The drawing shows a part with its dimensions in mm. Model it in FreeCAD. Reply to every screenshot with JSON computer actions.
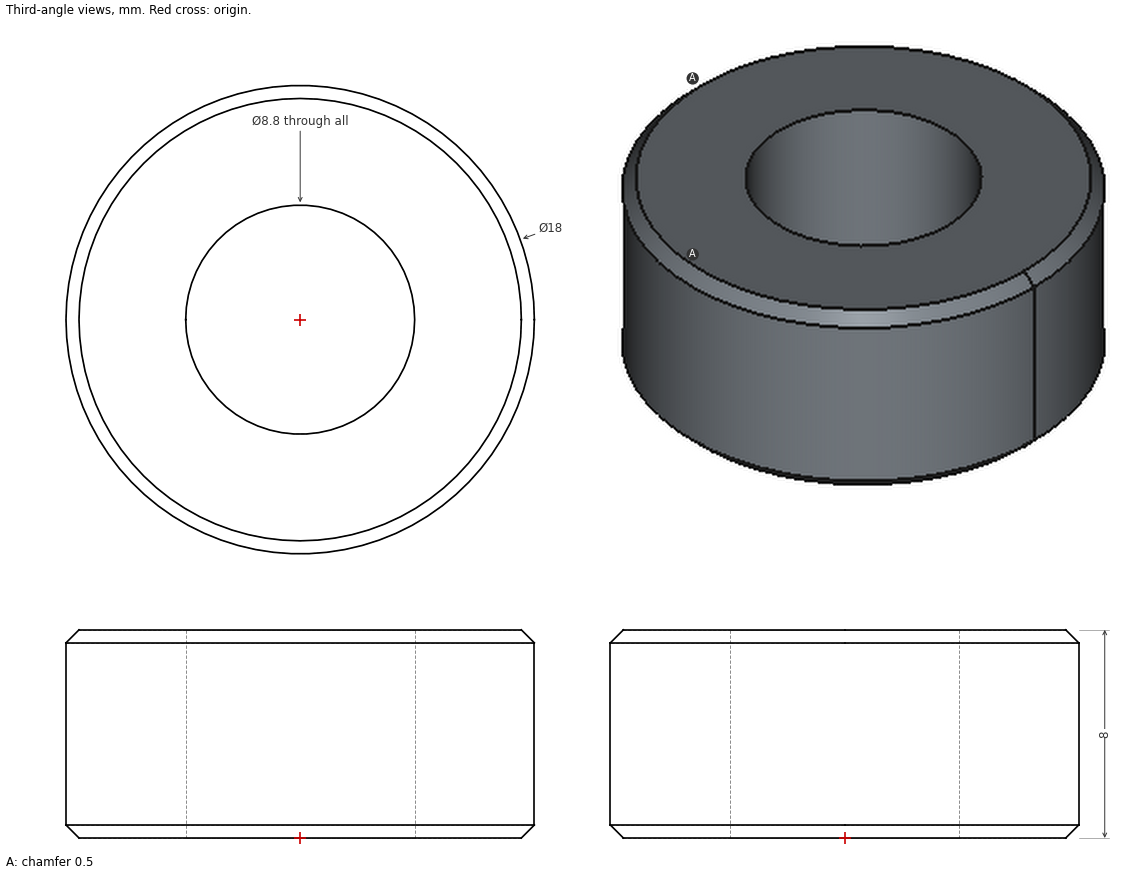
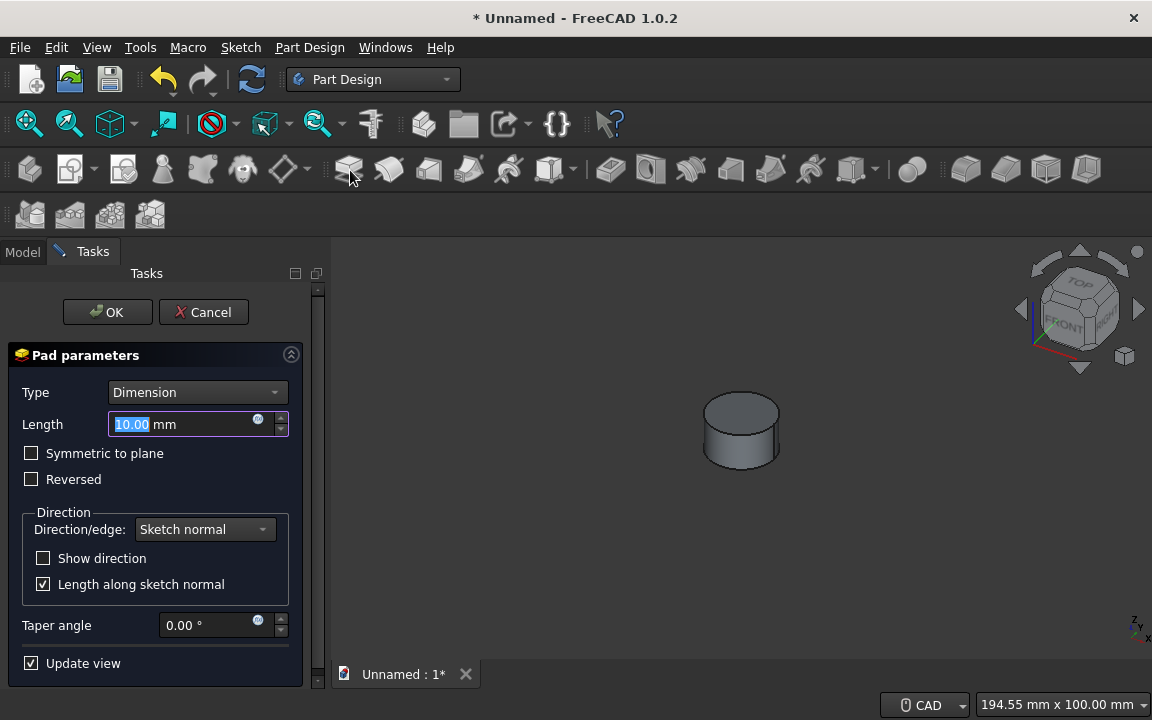
{"action": "type", "text": "8"}
{"action": "key", "text": "Tab"}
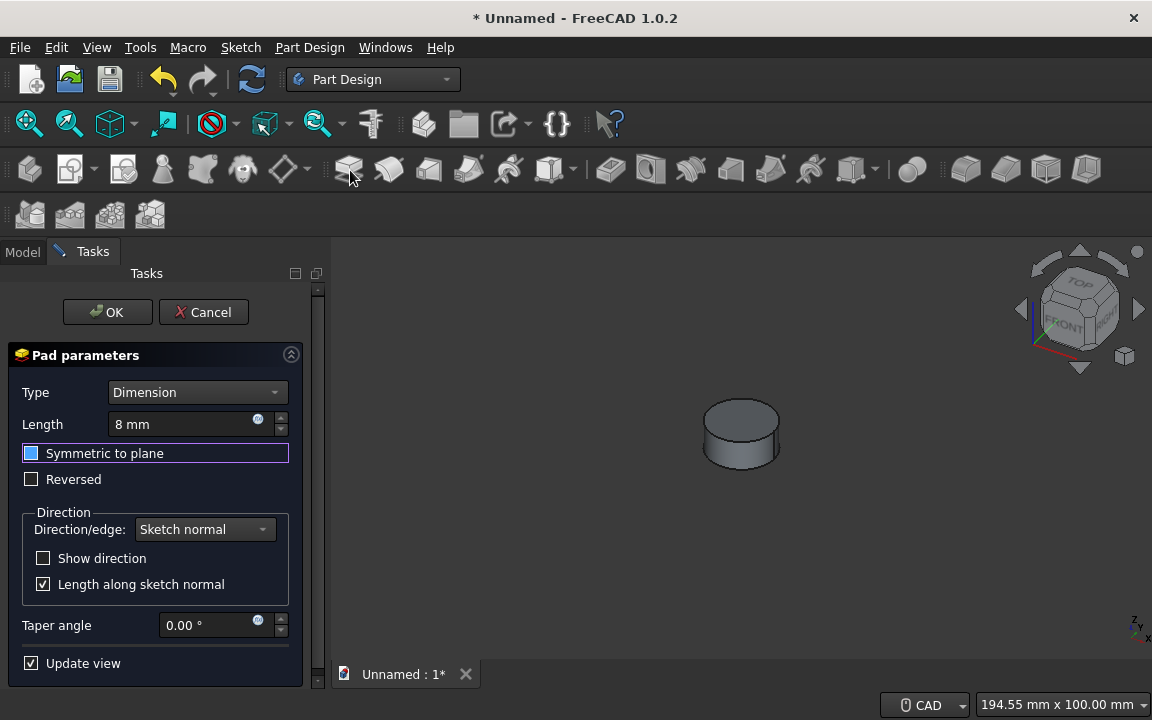
{"action": "left_click", "coordinate": [108, 312]}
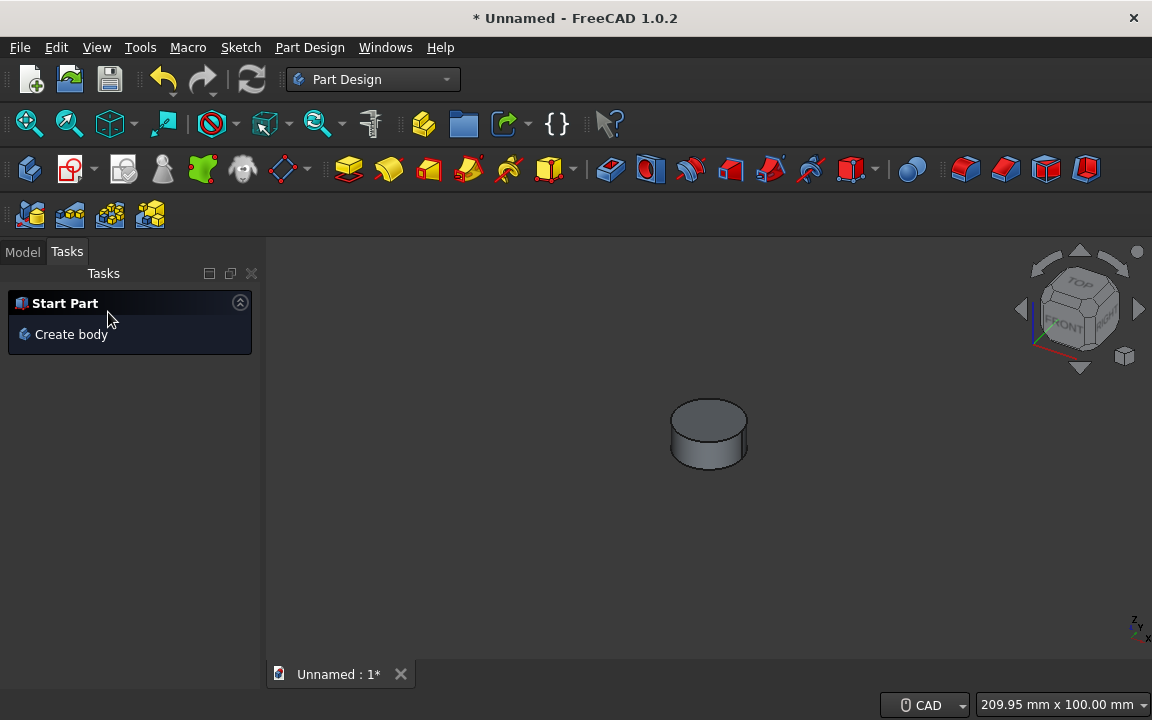
{"action": "key", "text": "v f"}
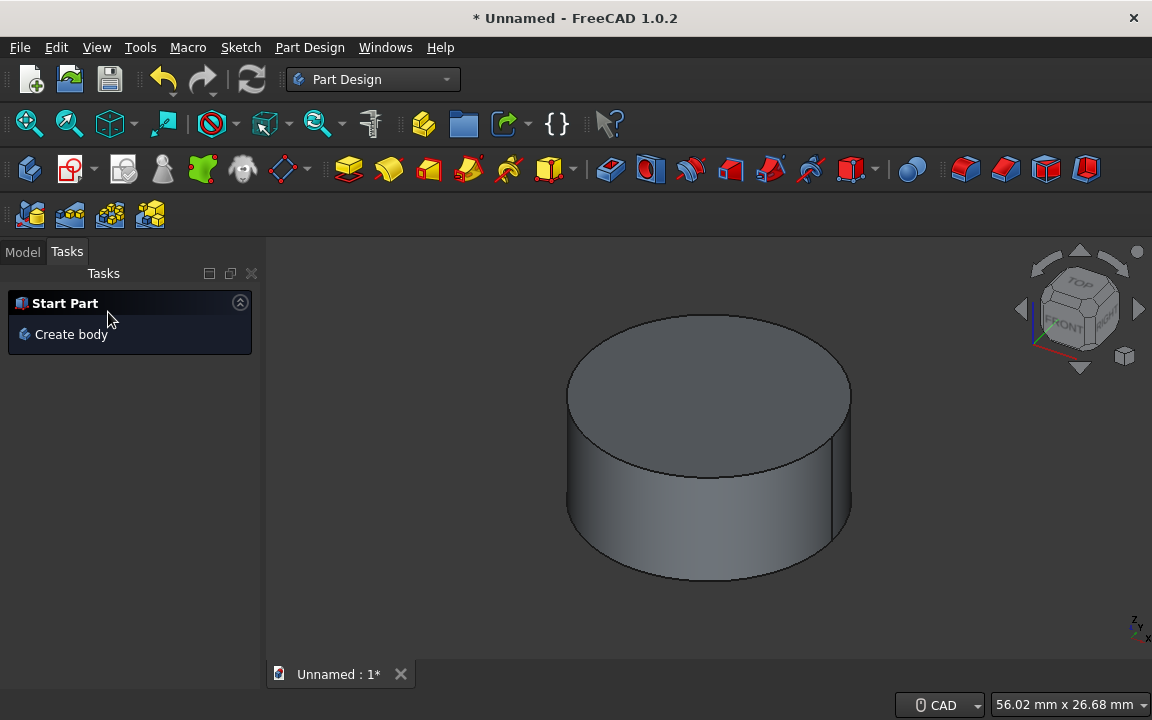
{"action": "left_click", "coordinate": [709, 395]}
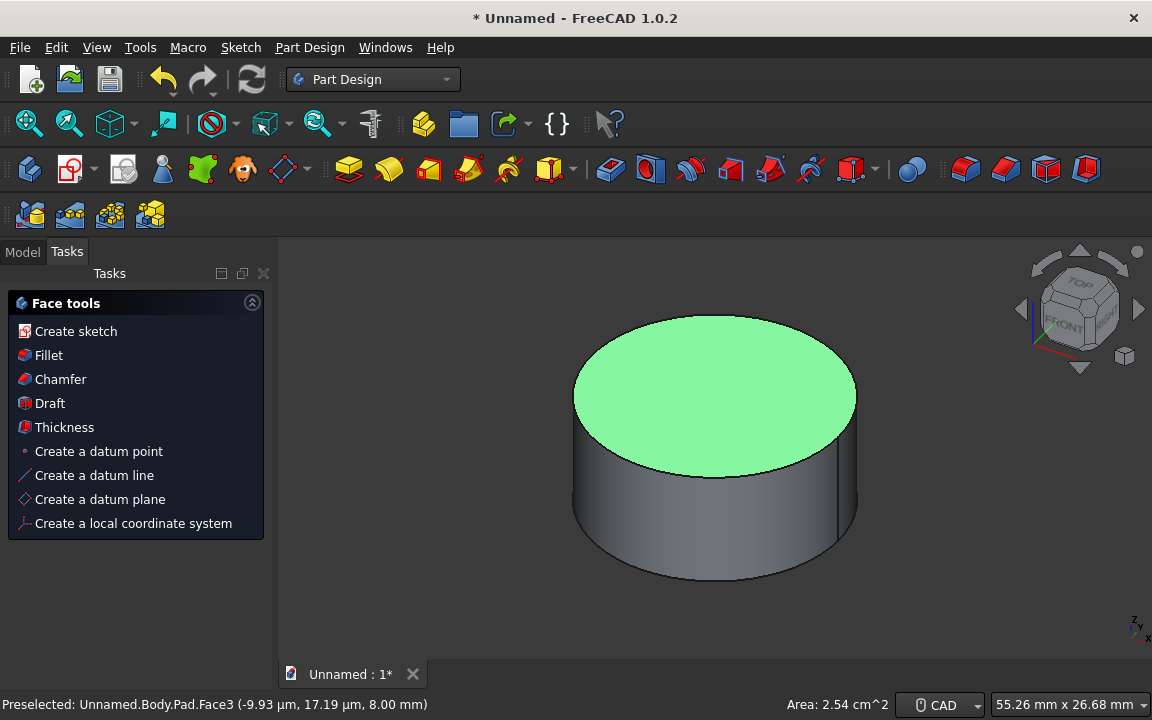
{"action": "left_click", "coordinate": [70, 170]}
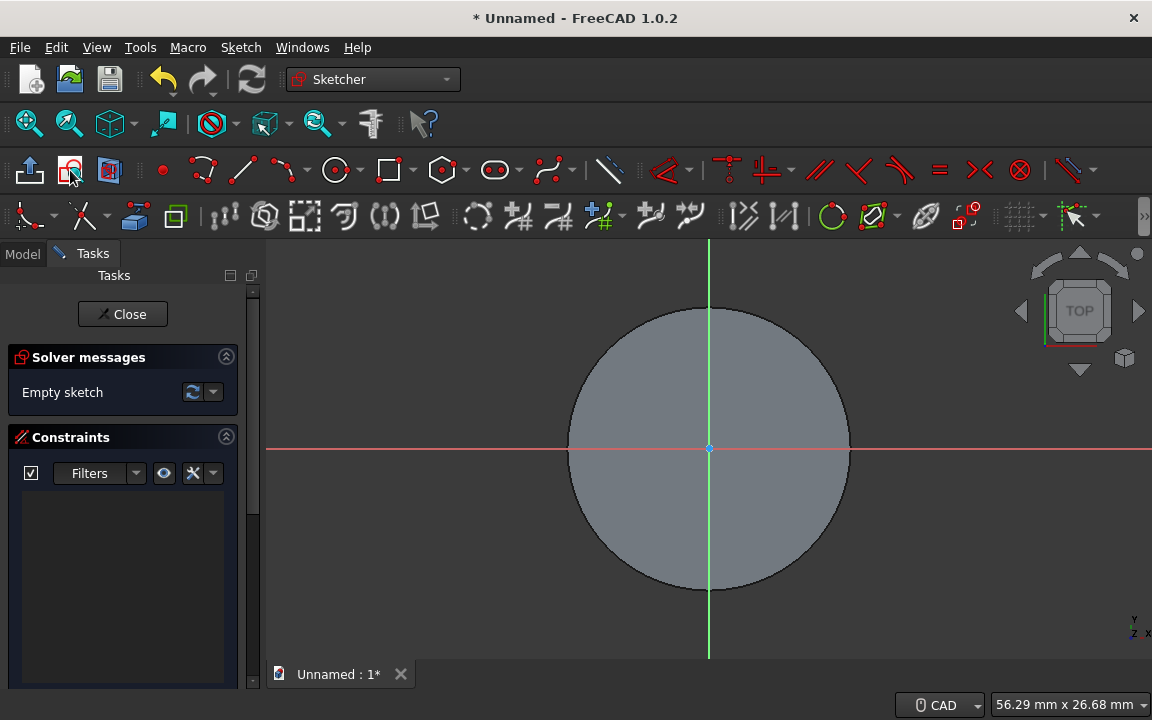
{"action": "scroll", "coordinate": [792, 449], "scroll_direction": "up", "scroll_amount": 3}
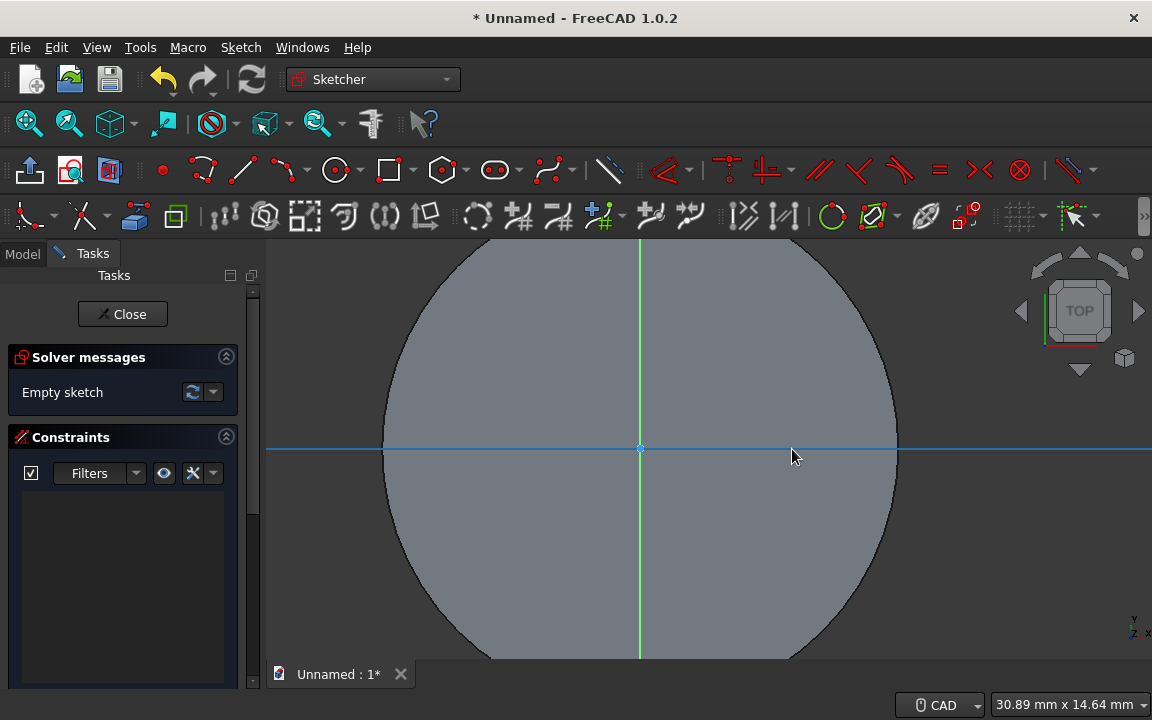
{"action": "key", "text": "g c"}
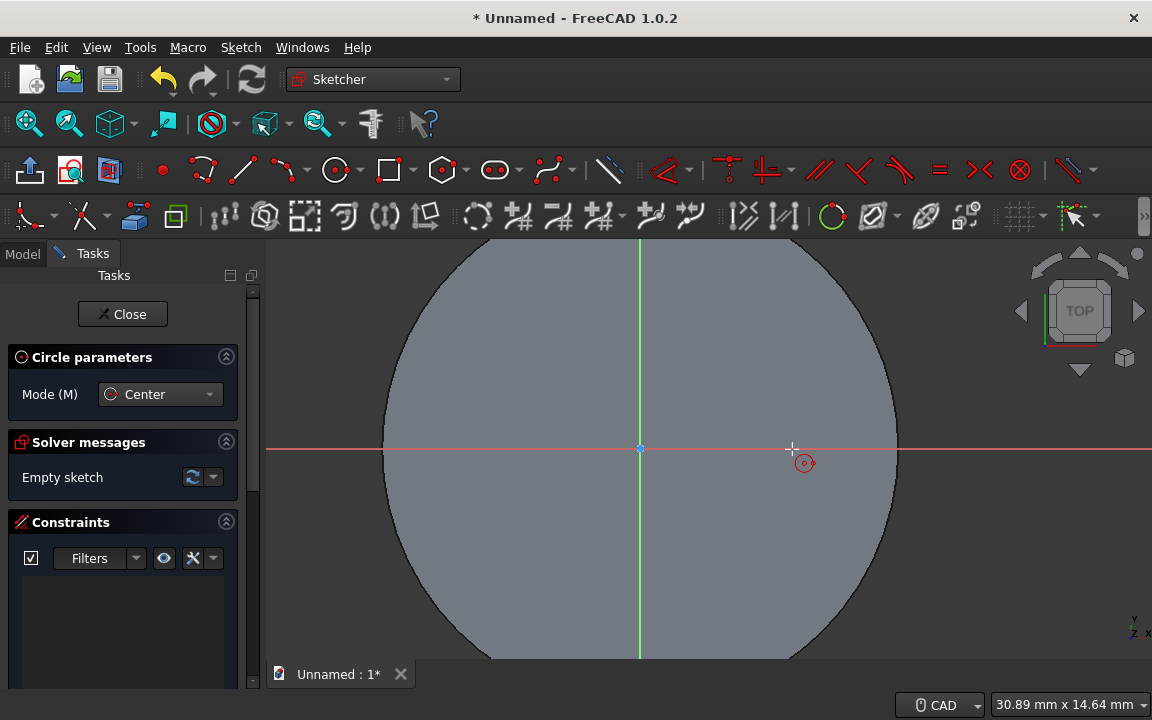
{"action": "left_click", "coordinate": [640, 449]}
{"action": "left_click", "coordinate": [730, 359]}
{"action": "key", "text": "Escape"}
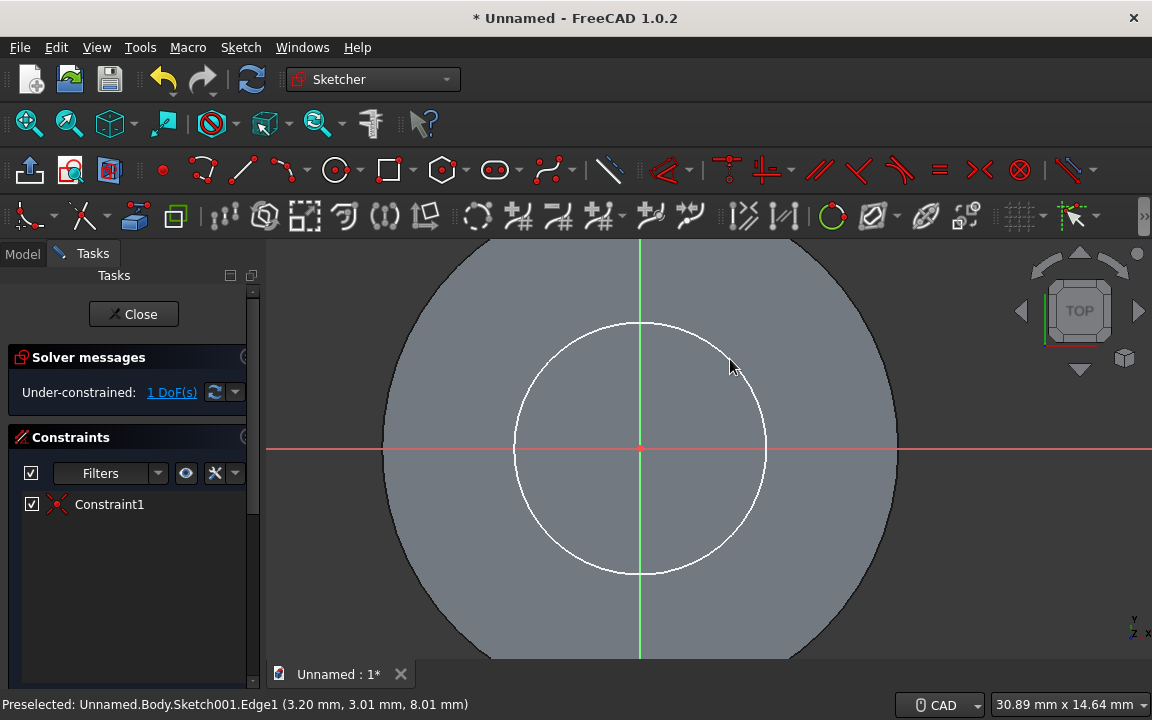
{"action": "left_click", "coordinate": [664, 170]}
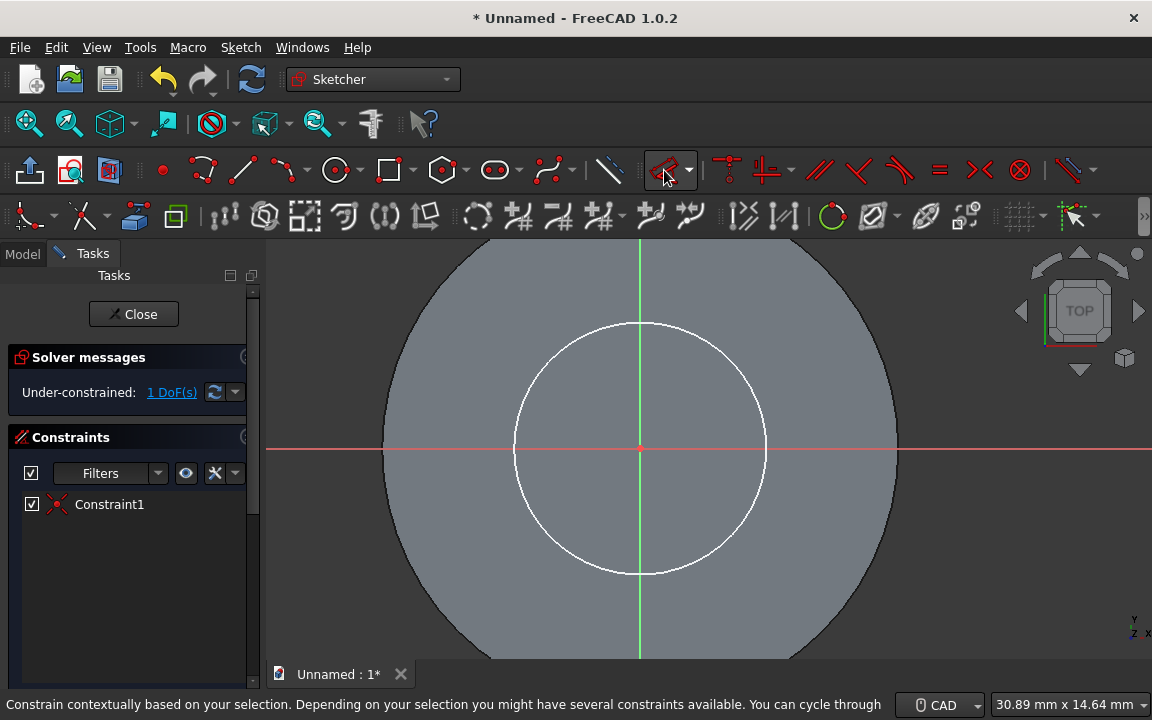
{"action": "left_click", "coordinate": [729, 359]}
{"action": "left_click", "coordinate": [752, 336]}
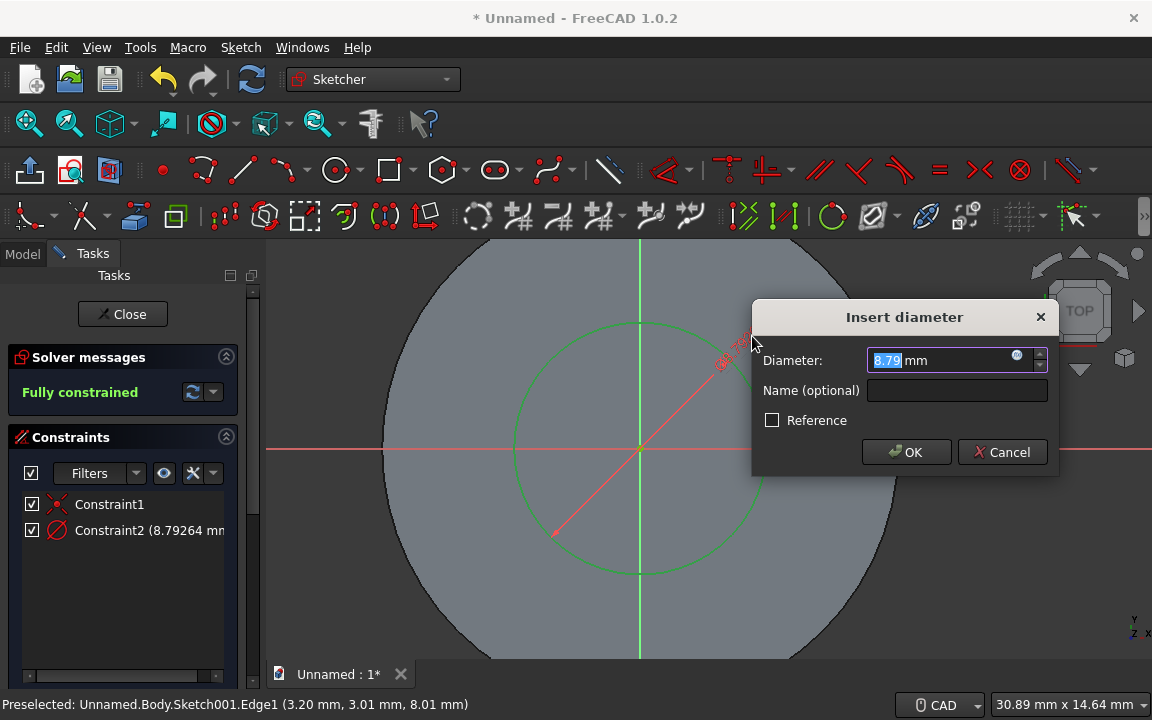
{"action": "type", "text": "8.8"}
{"action": "key", "text": "Return"}
{"action": "key", "text": "Escape"}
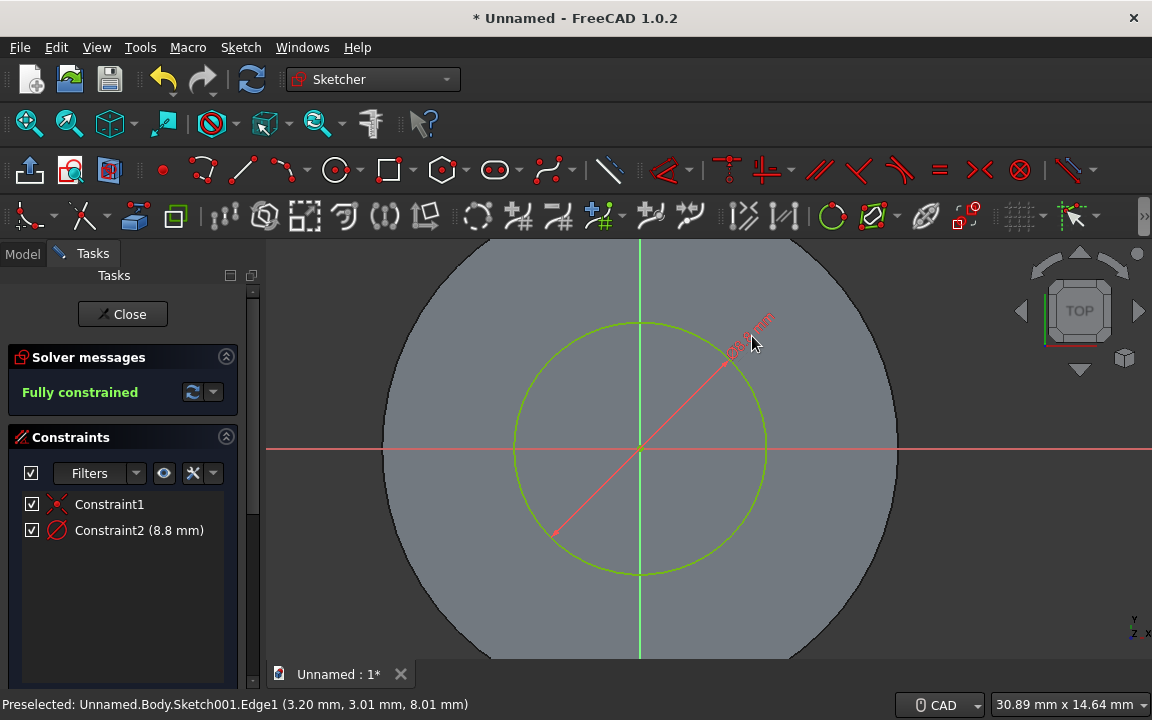
{"action": "left_click", "coordinate": [123, 314]}